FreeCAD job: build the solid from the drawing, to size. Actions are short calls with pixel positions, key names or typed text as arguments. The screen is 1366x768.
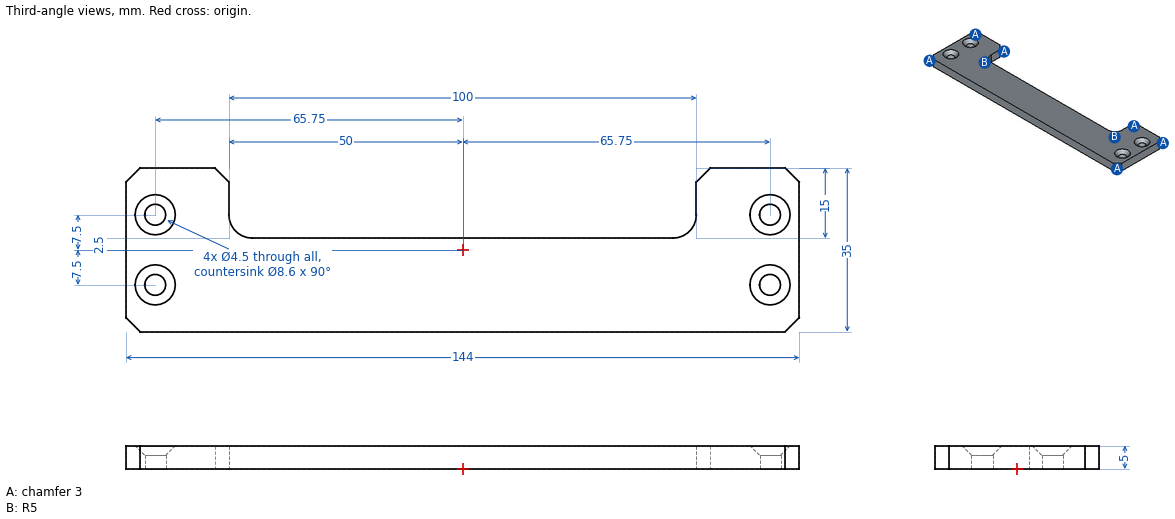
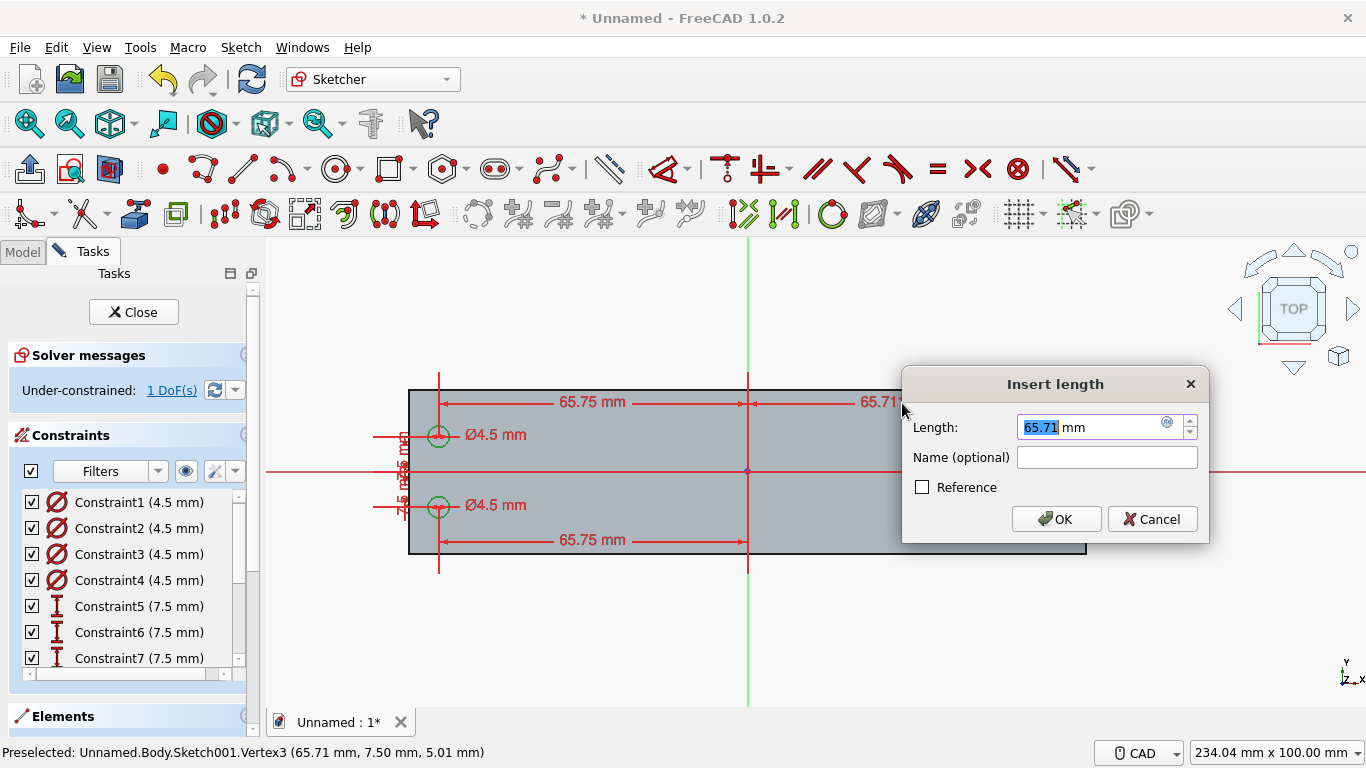
text(65.75)
key(Return)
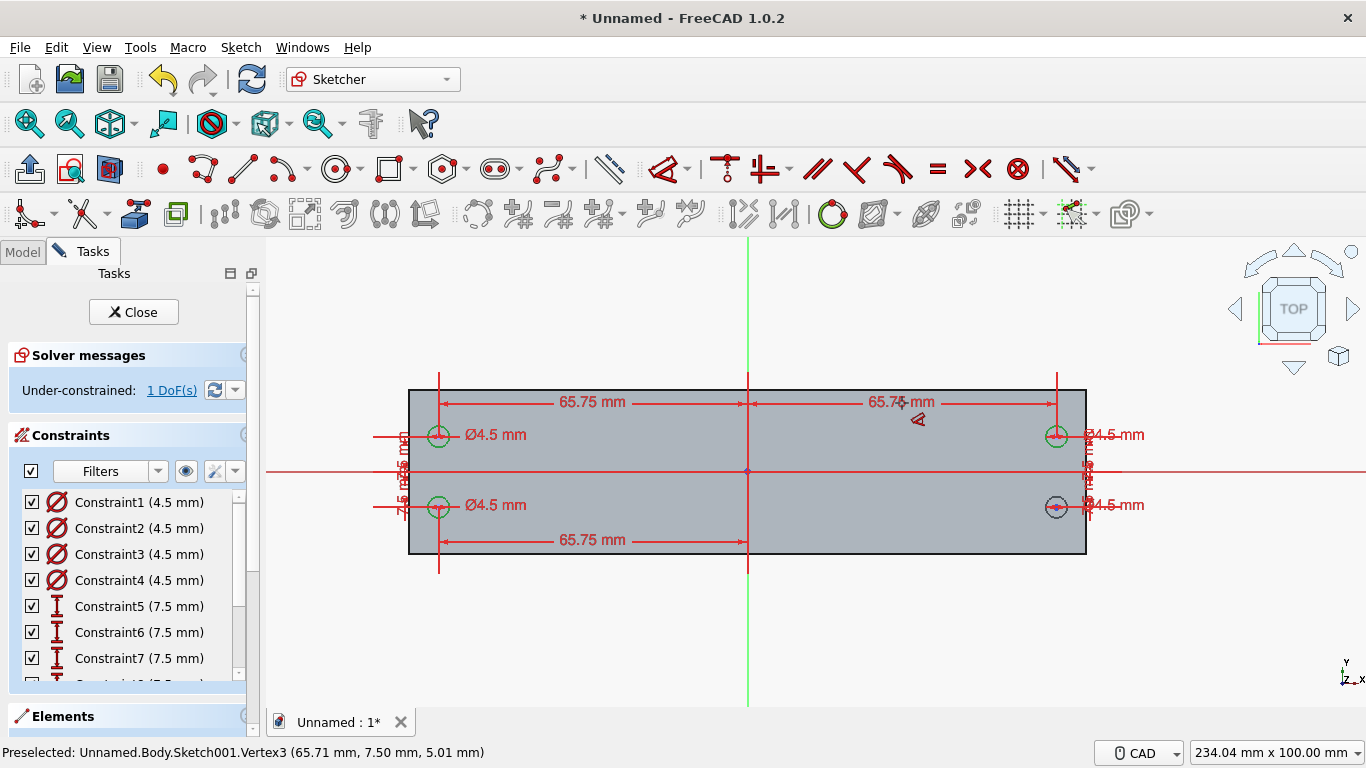
click(1056, 507)
click(902, 541)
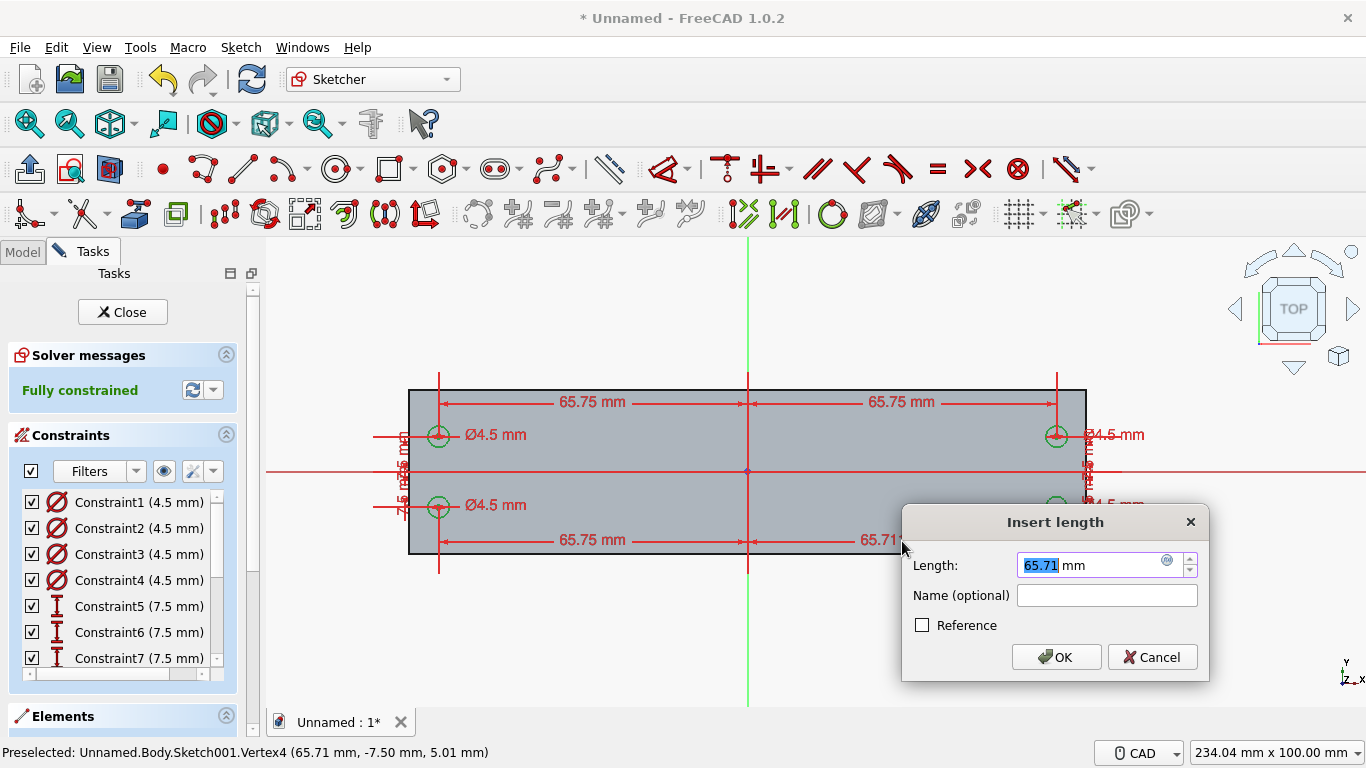
text(65.75)
key(Return)
key(Escape)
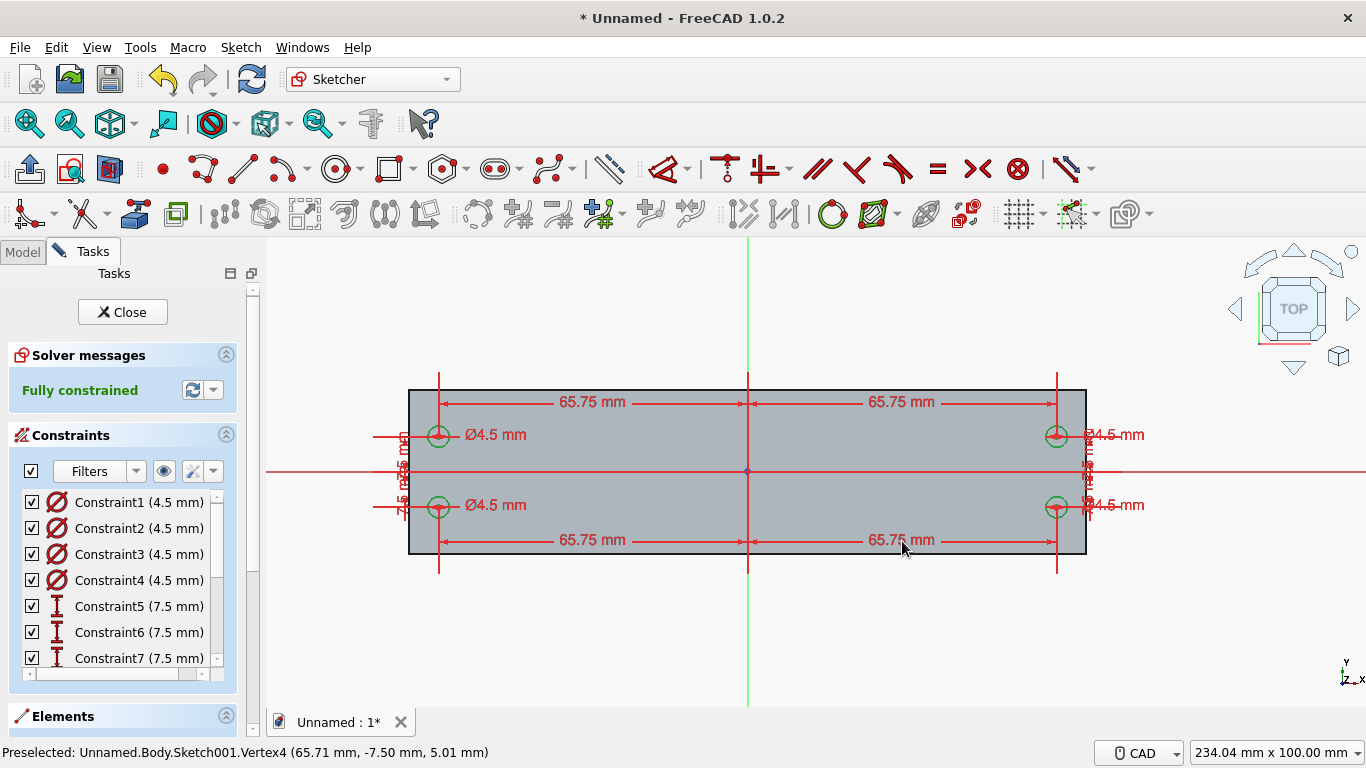
click(123, 312)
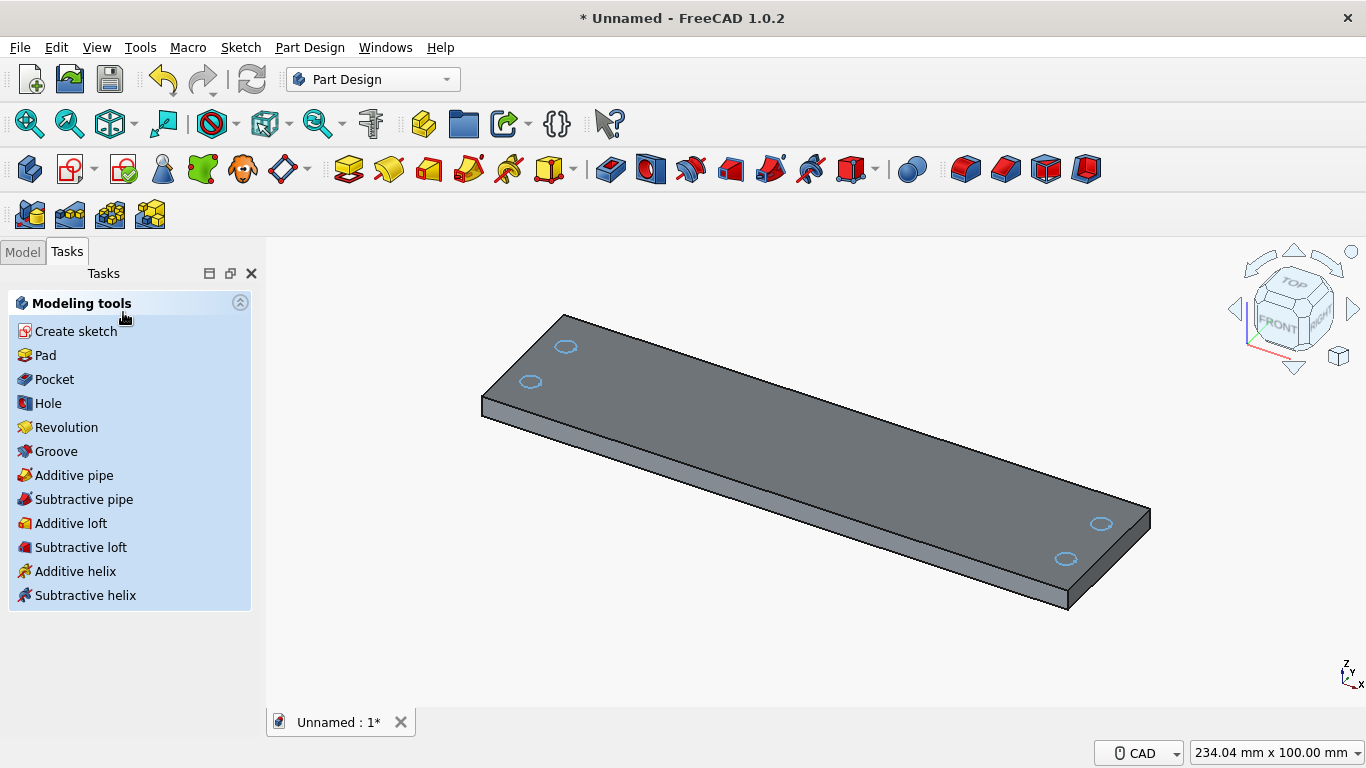
click(652, 170)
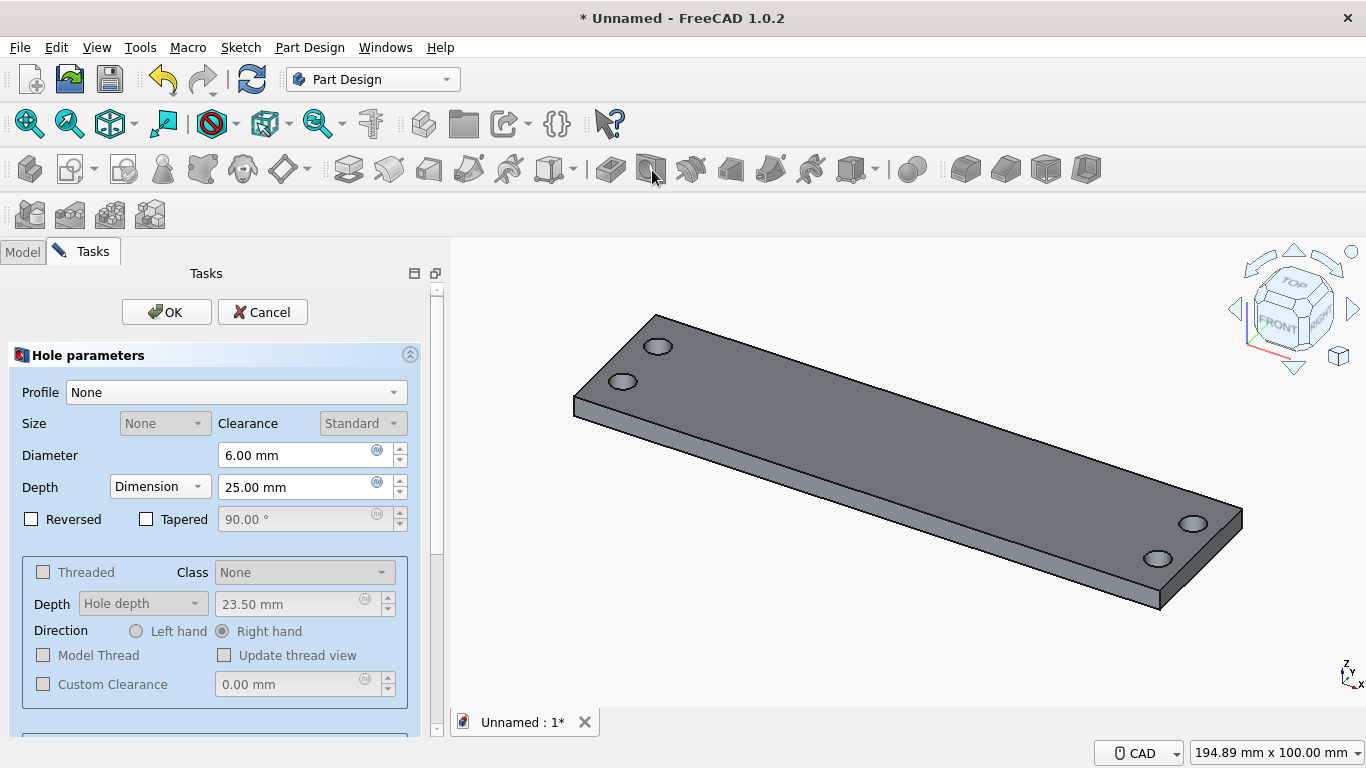
triple_click(305, 455)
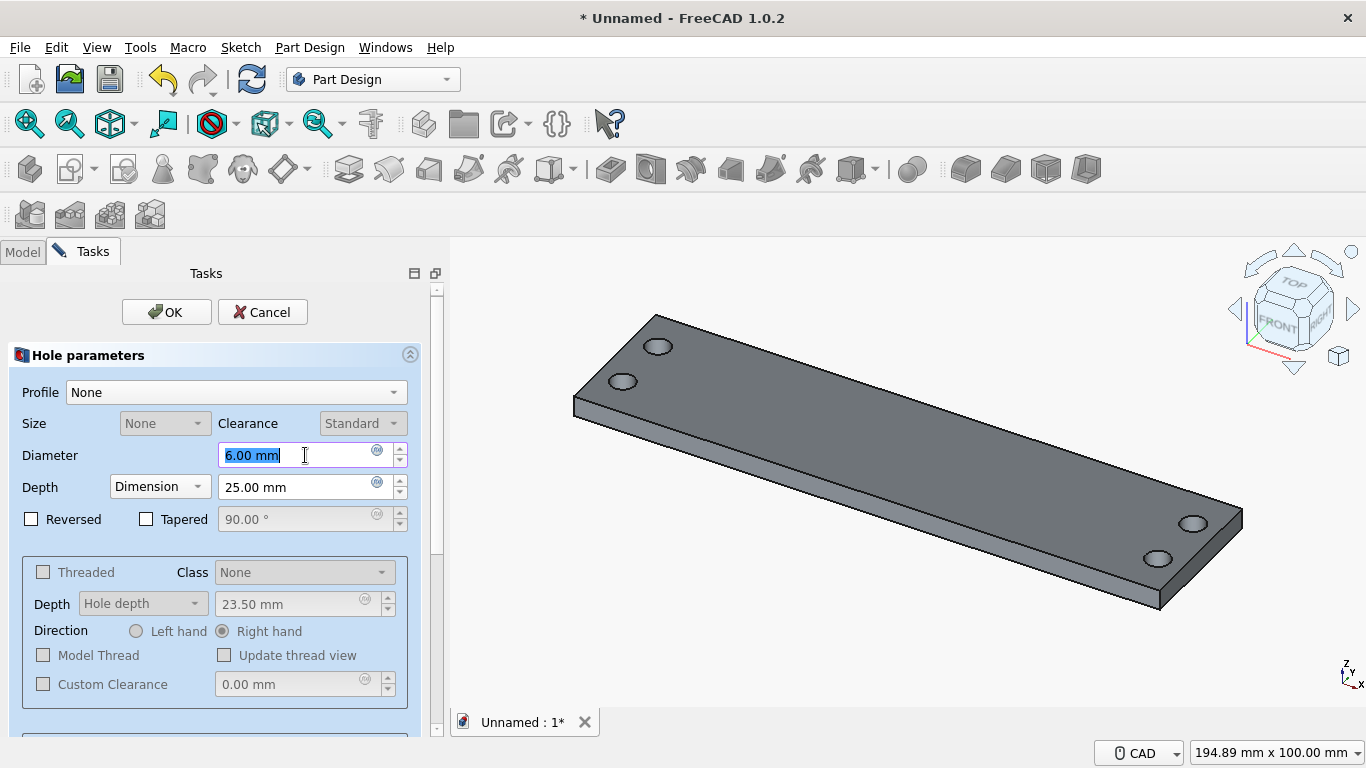
text(4.5)
key(Tab)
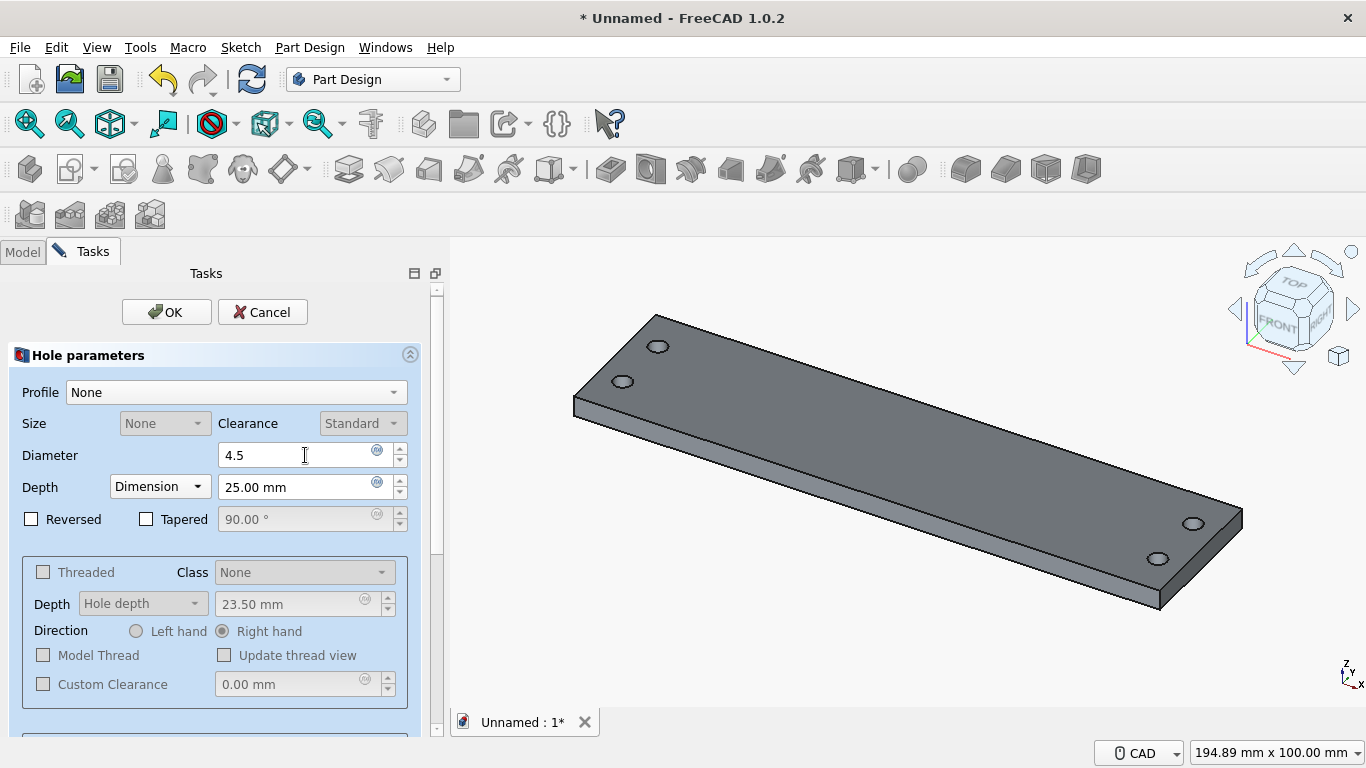
click(161, 486)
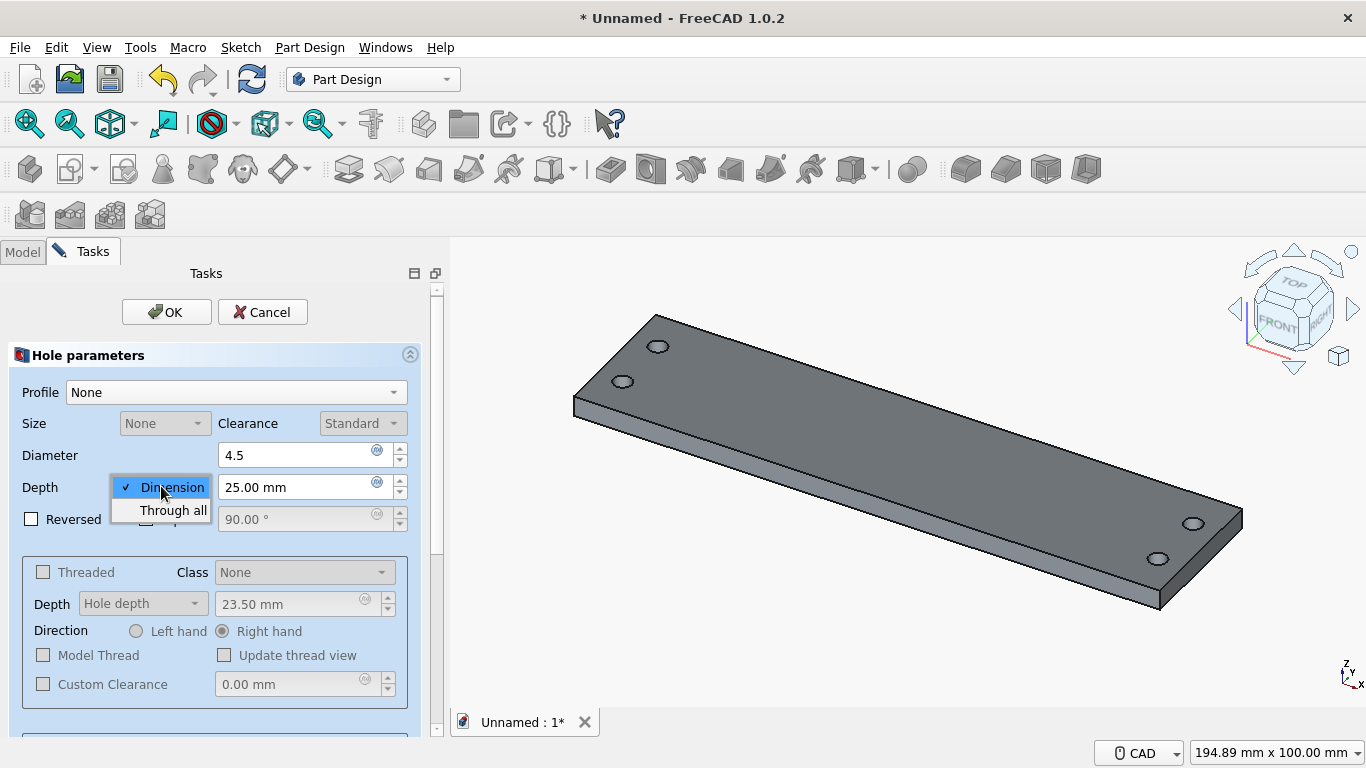
click(160, 510)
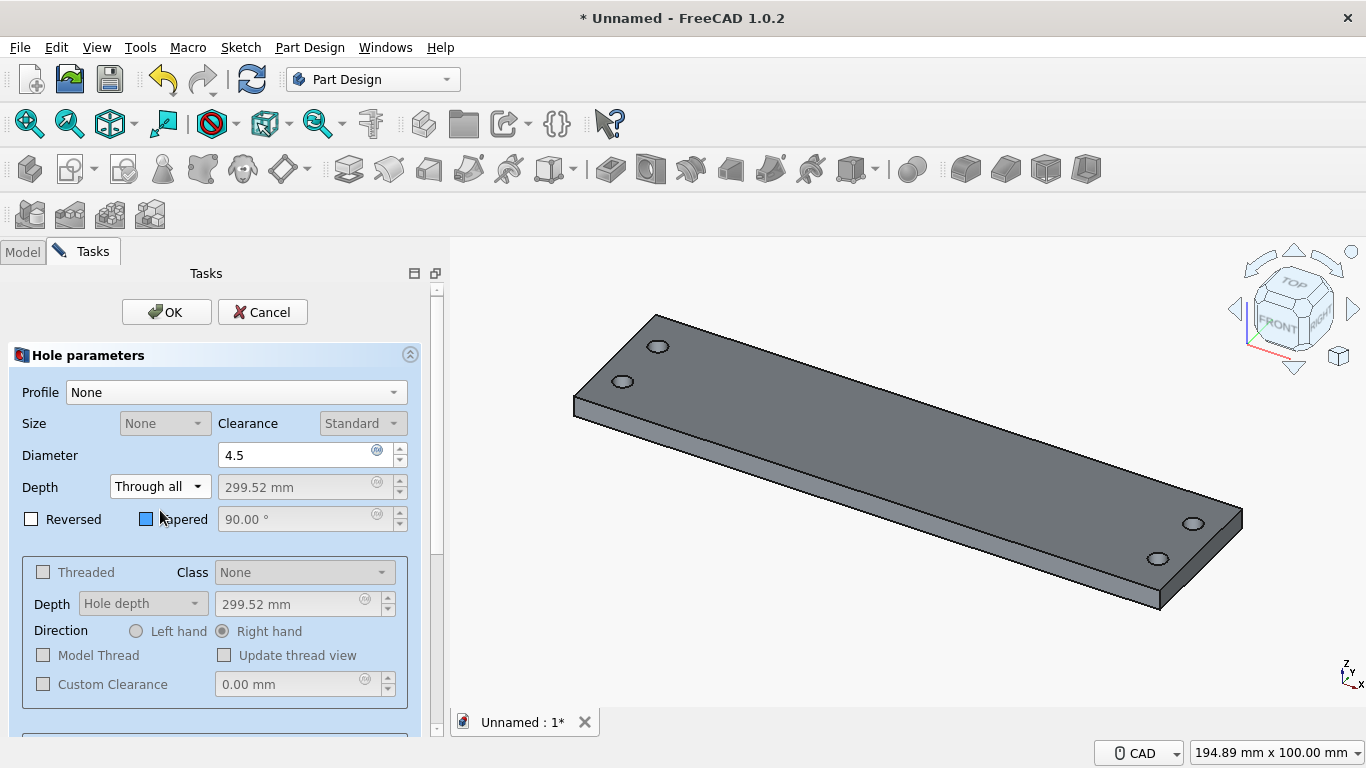
scroll(437, 510, down, 2)